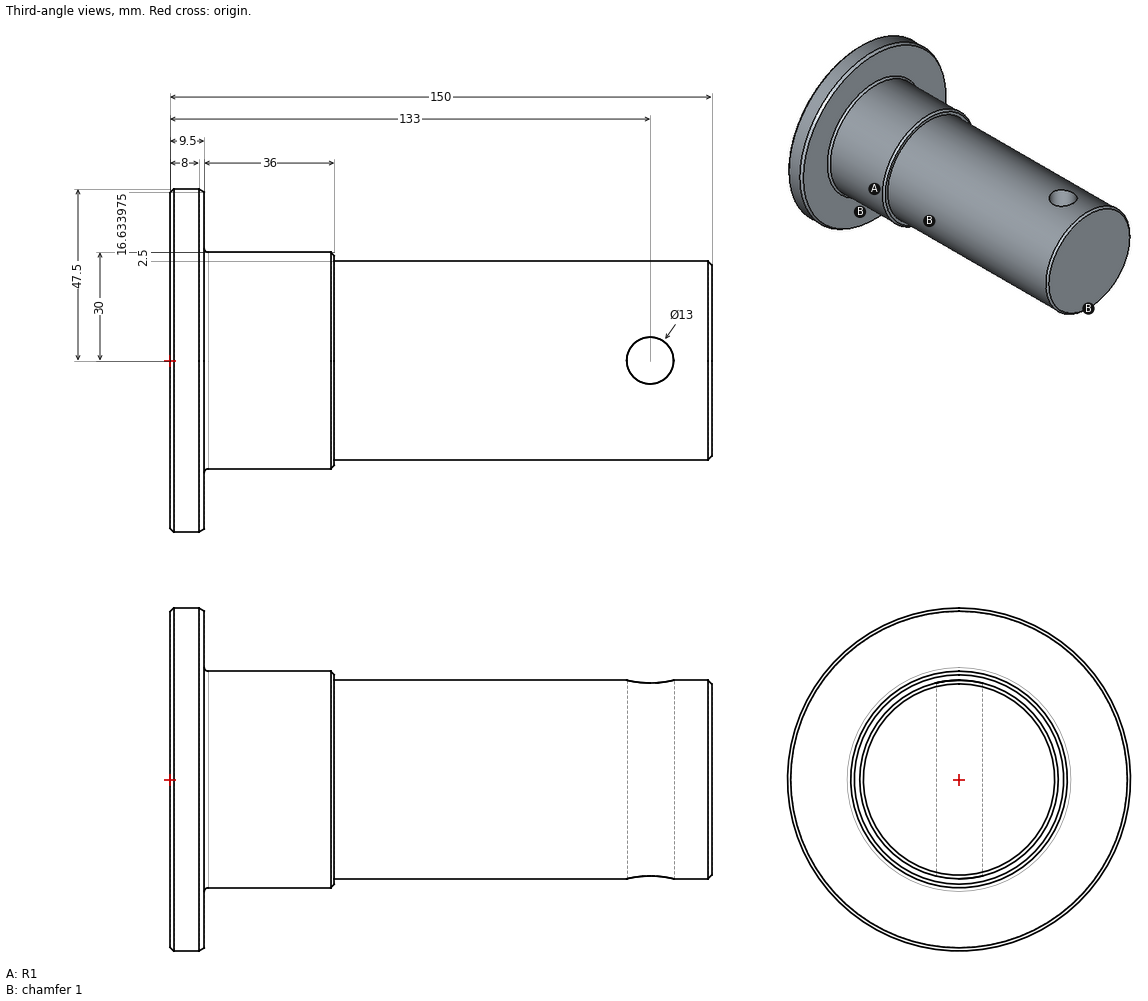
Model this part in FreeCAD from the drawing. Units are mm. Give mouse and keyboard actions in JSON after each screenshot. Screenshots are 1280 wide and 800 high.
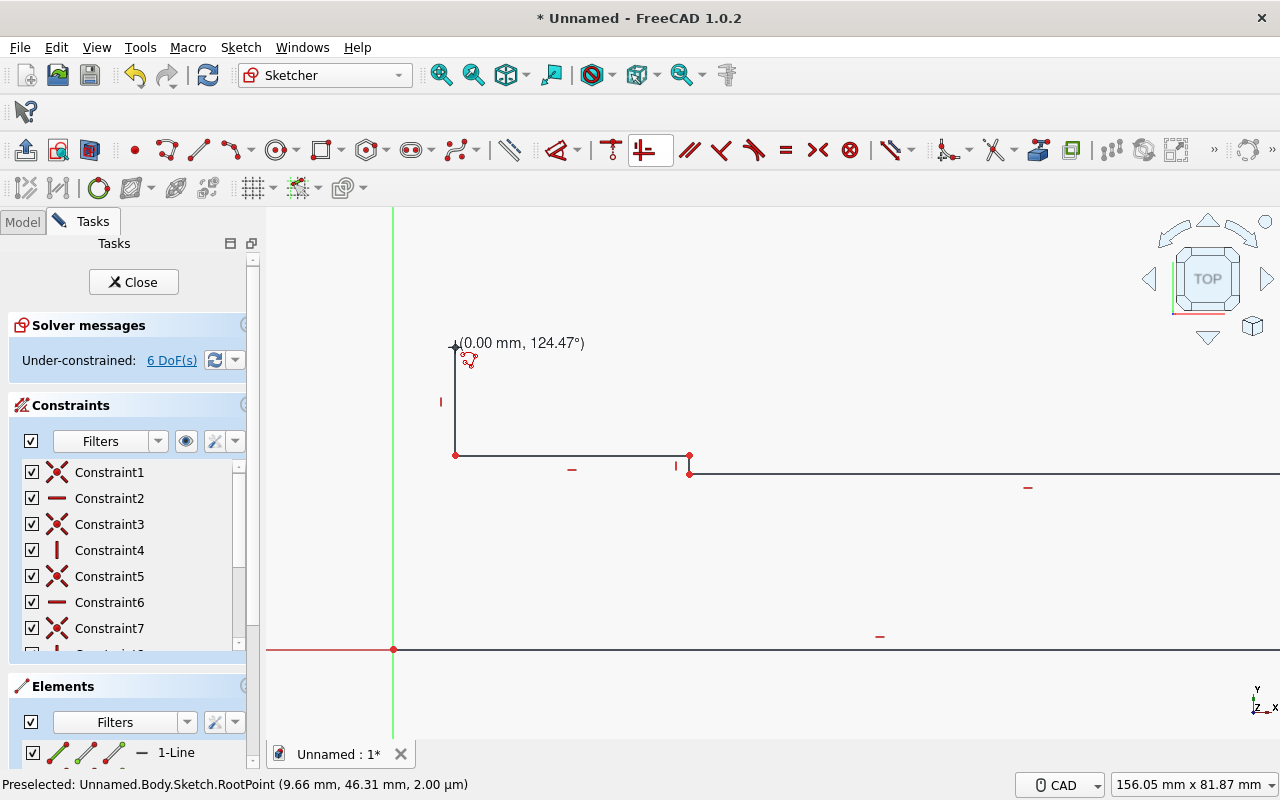
{"action": "scroll", "coordinate": [445, 341], "scroll_direction": "up", "scroll_amount": 2}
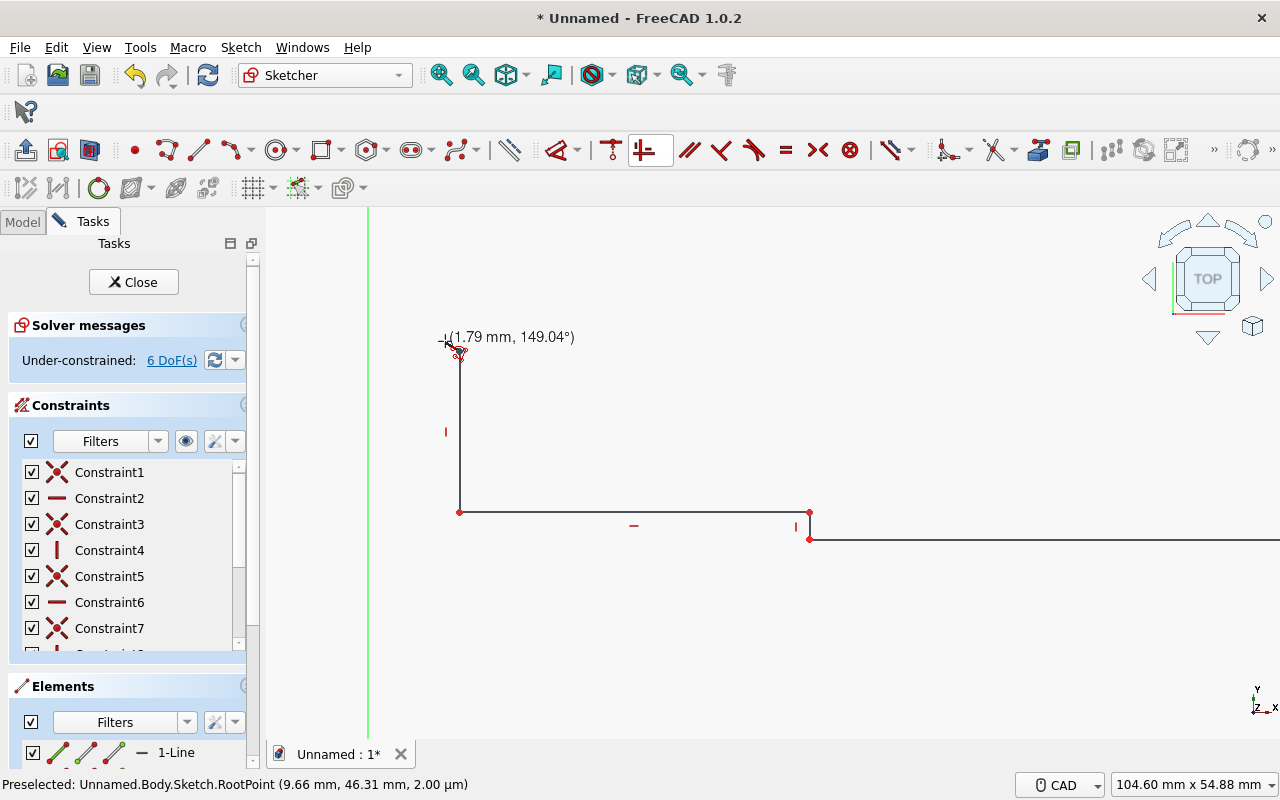
{"action": "left_click", "coordinate": [445, 341]}
{"action": "left_click", "coordinate": [377, 341]}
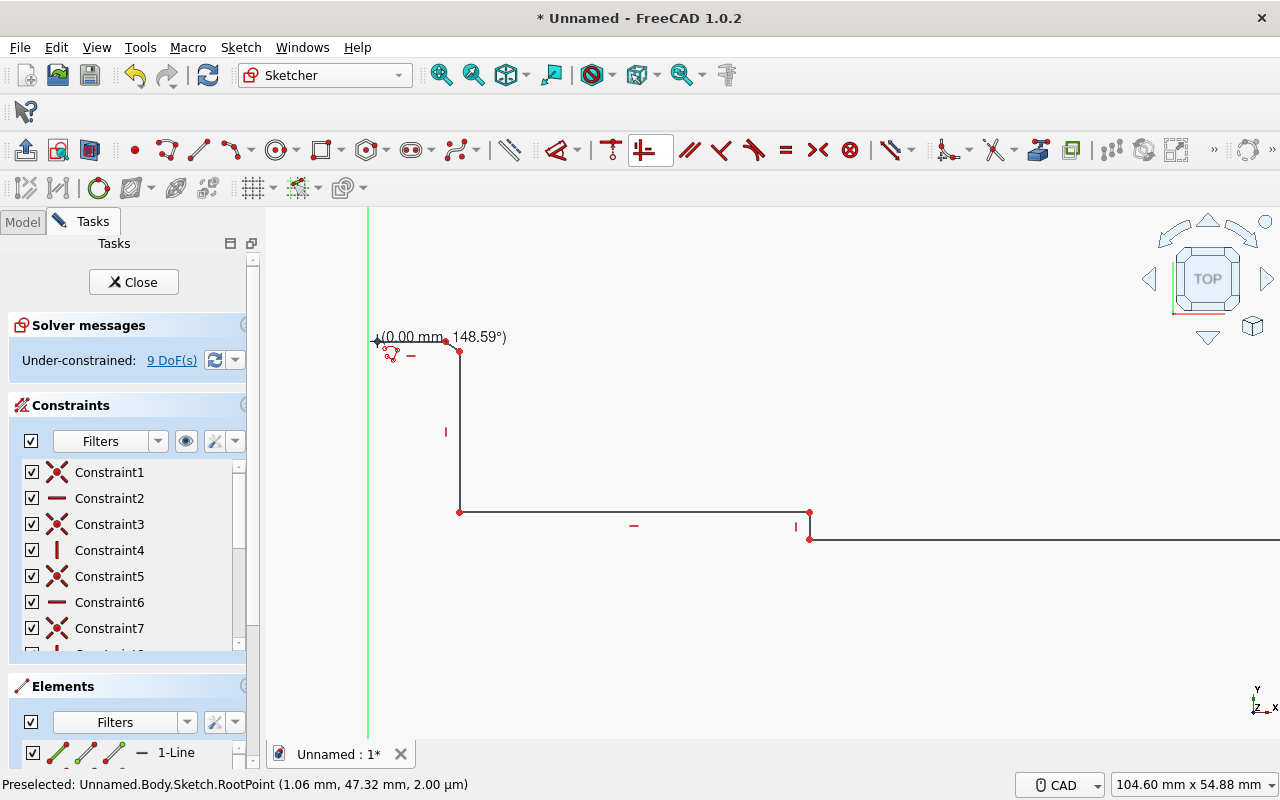
{"action": "scroll", "coordinate": [477, 416], "scroll_direction": "down", "scroll_amount": 5}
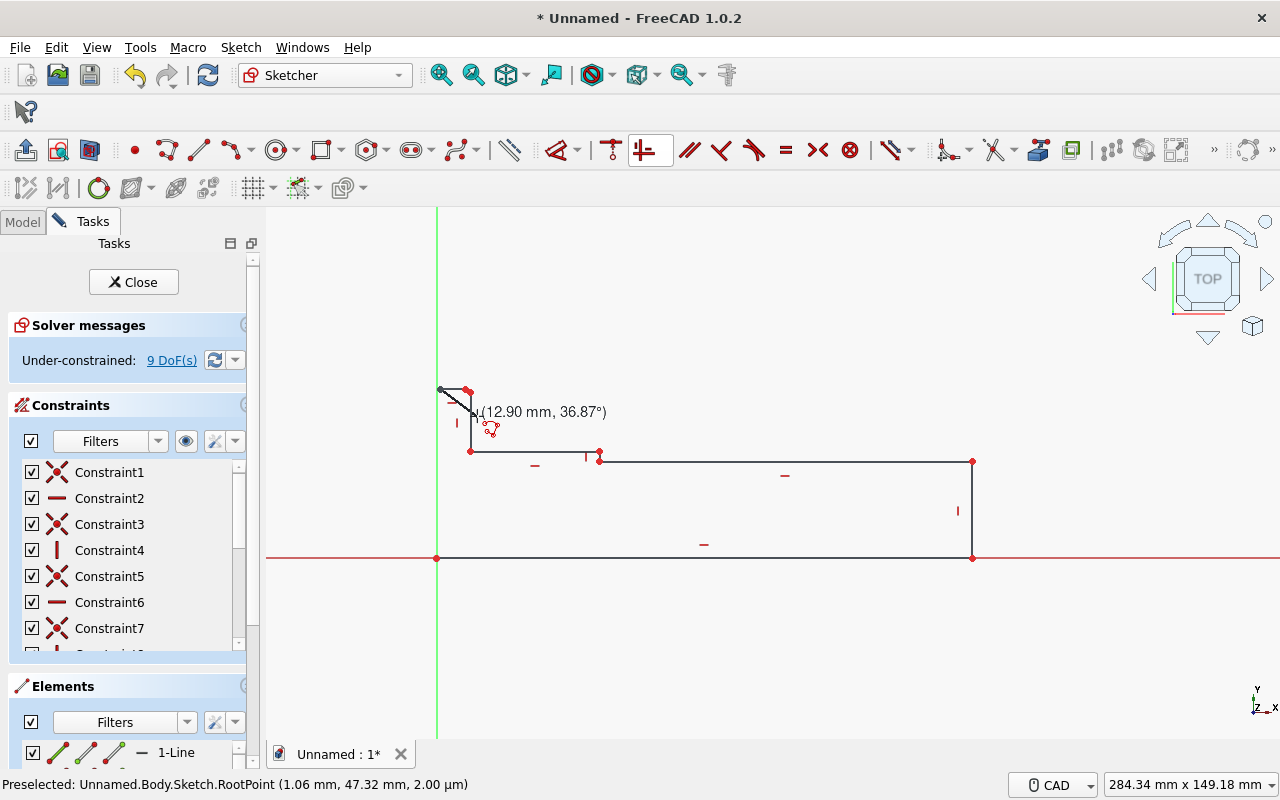
{"action": "left_click", "coordinate": [437, 558]}
{"action": "key", "text": "Escape"}
{"action": "key", "text": "Escape"}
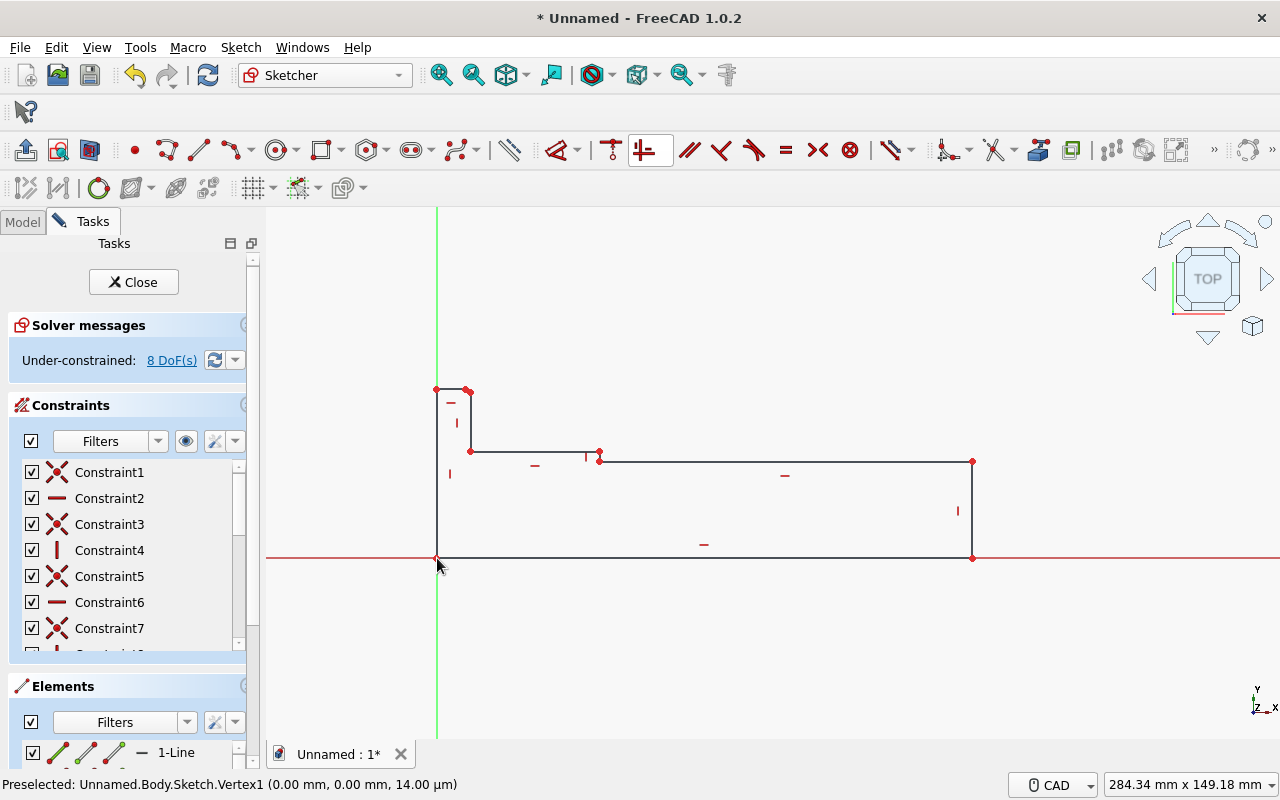
{"action": "key", "text": "d"}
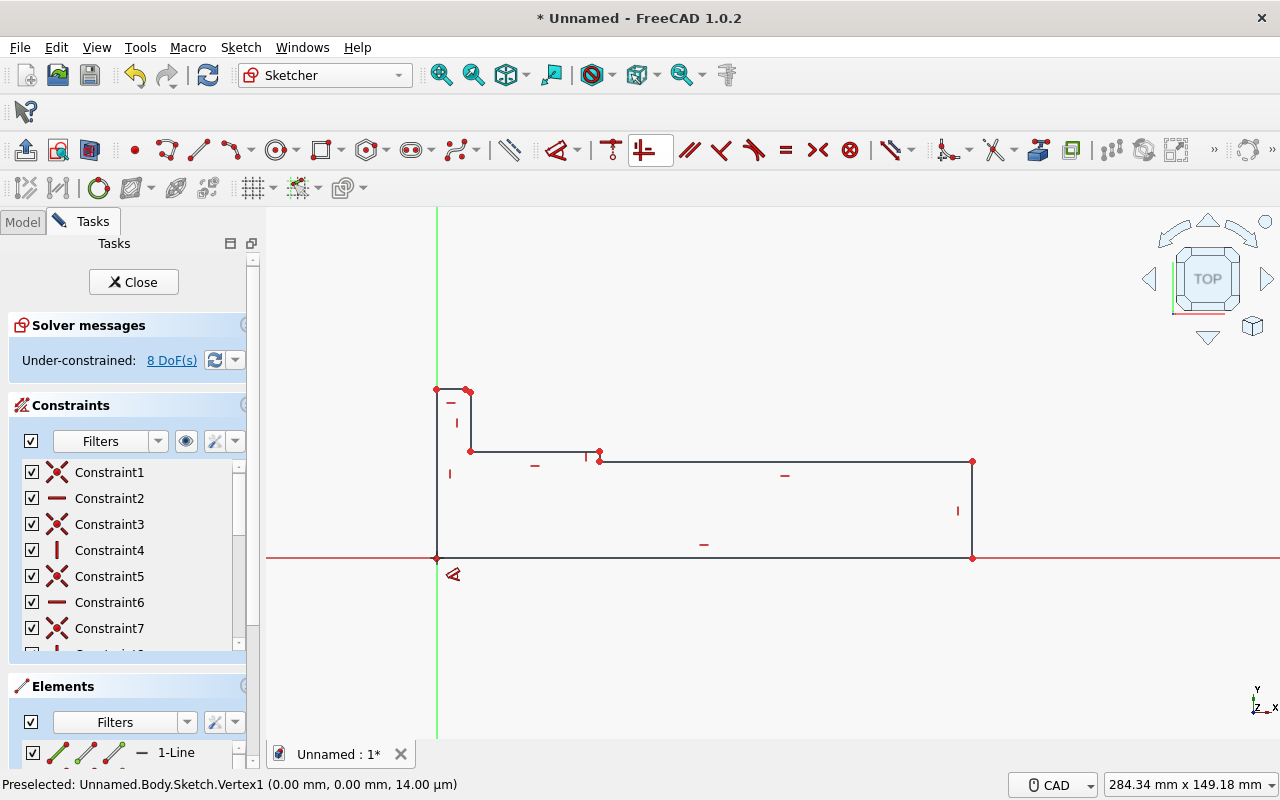
{"action": "scroll", "coordinate": [454, 389], "scroll_direction": "up", "scroll_amount": 2}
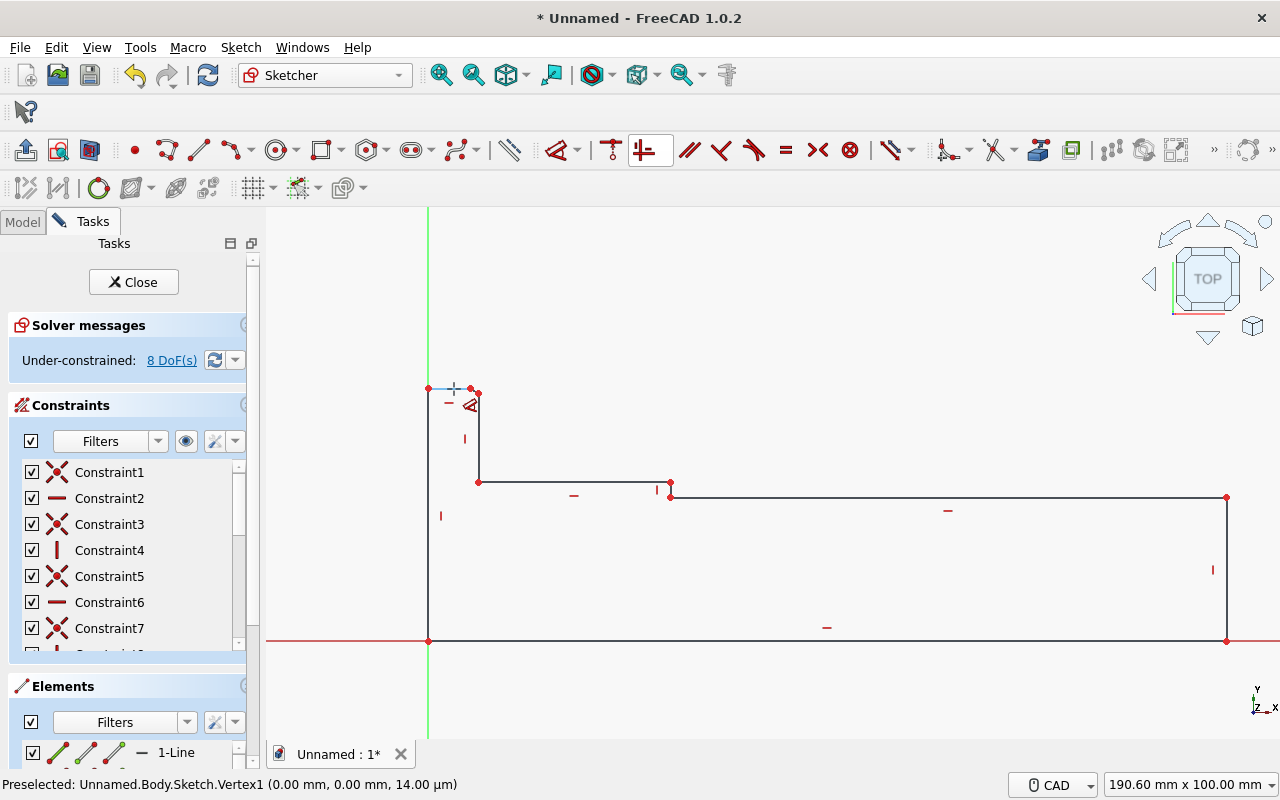
{"action": "left_click", "coordinate": [454, 389]}
{"action": "left_click", "coordinate": [450, 355]}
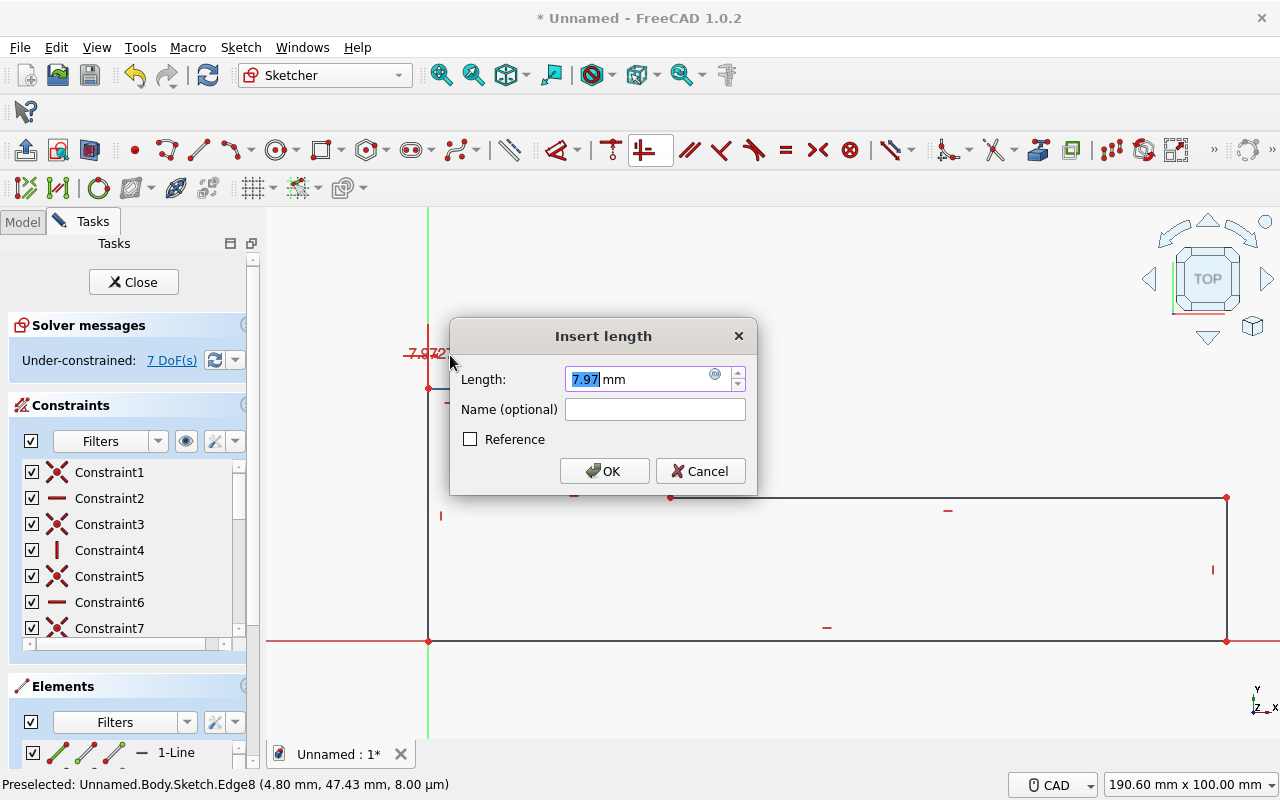
{"action": "type", "text": "8"}
{"action": "key", "text": "Return"}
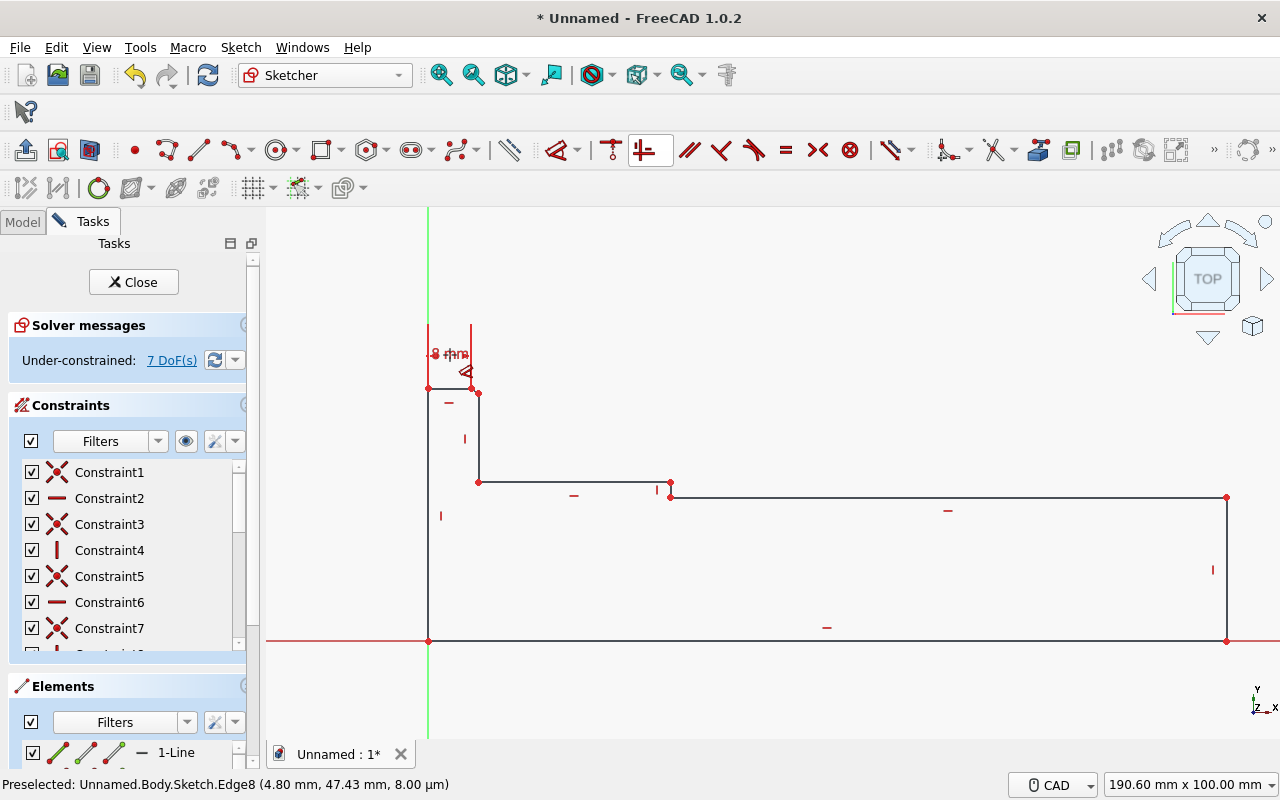
{"action": "left_click", "coordinate": [613, 482]}
{"action": "left_click", "coordinate": [575, 448]}